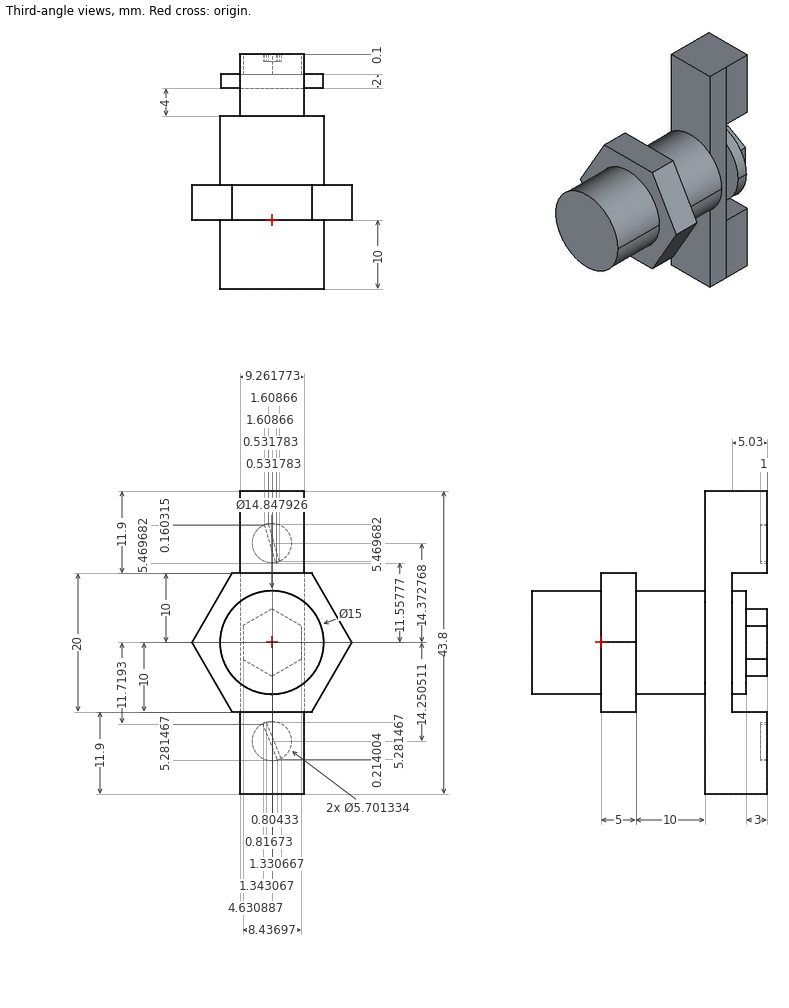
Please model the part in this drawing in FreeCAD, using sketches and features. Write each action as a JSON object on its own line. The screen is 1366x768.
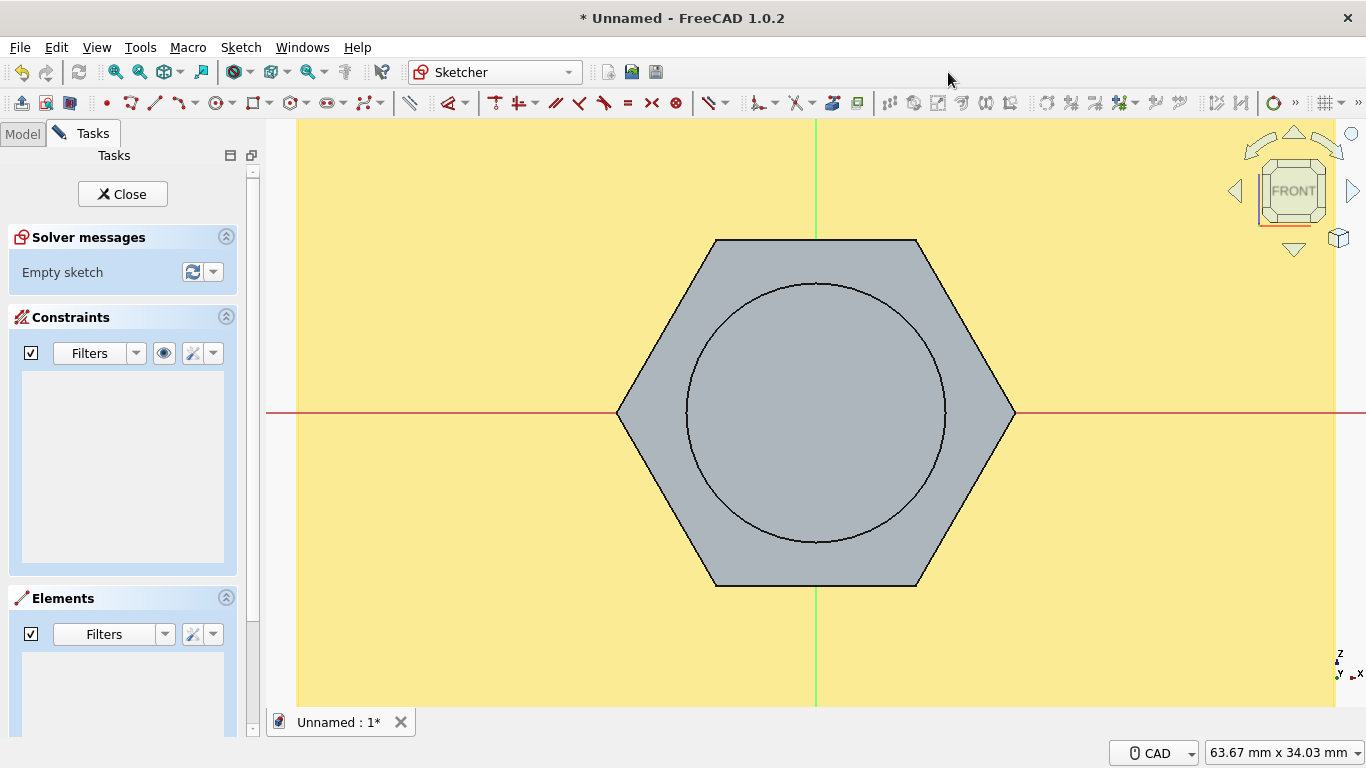
{"action": "left_click", "coordinate": [70, 104]}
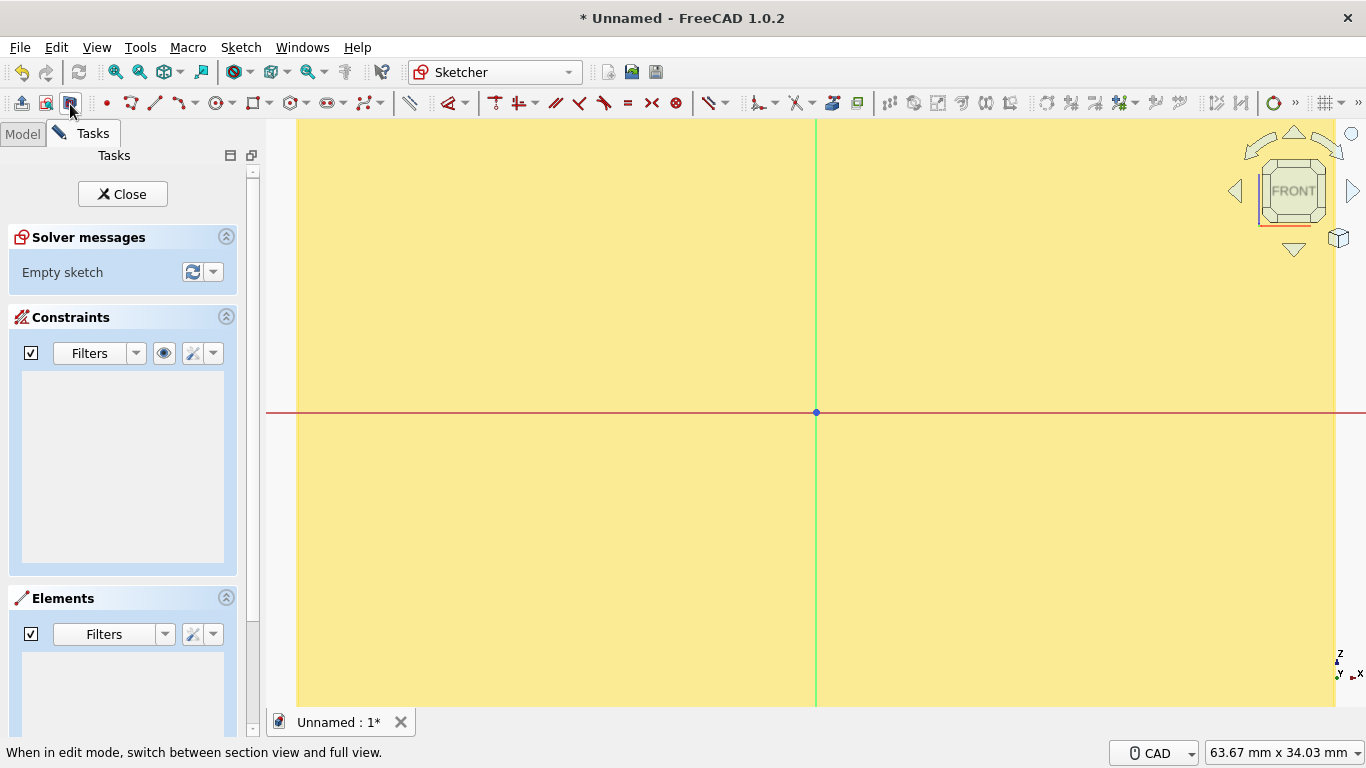
{"action": "scroll", "coordinate": [955, 413], "scroll_direction": "up", "scroll_amount": 2}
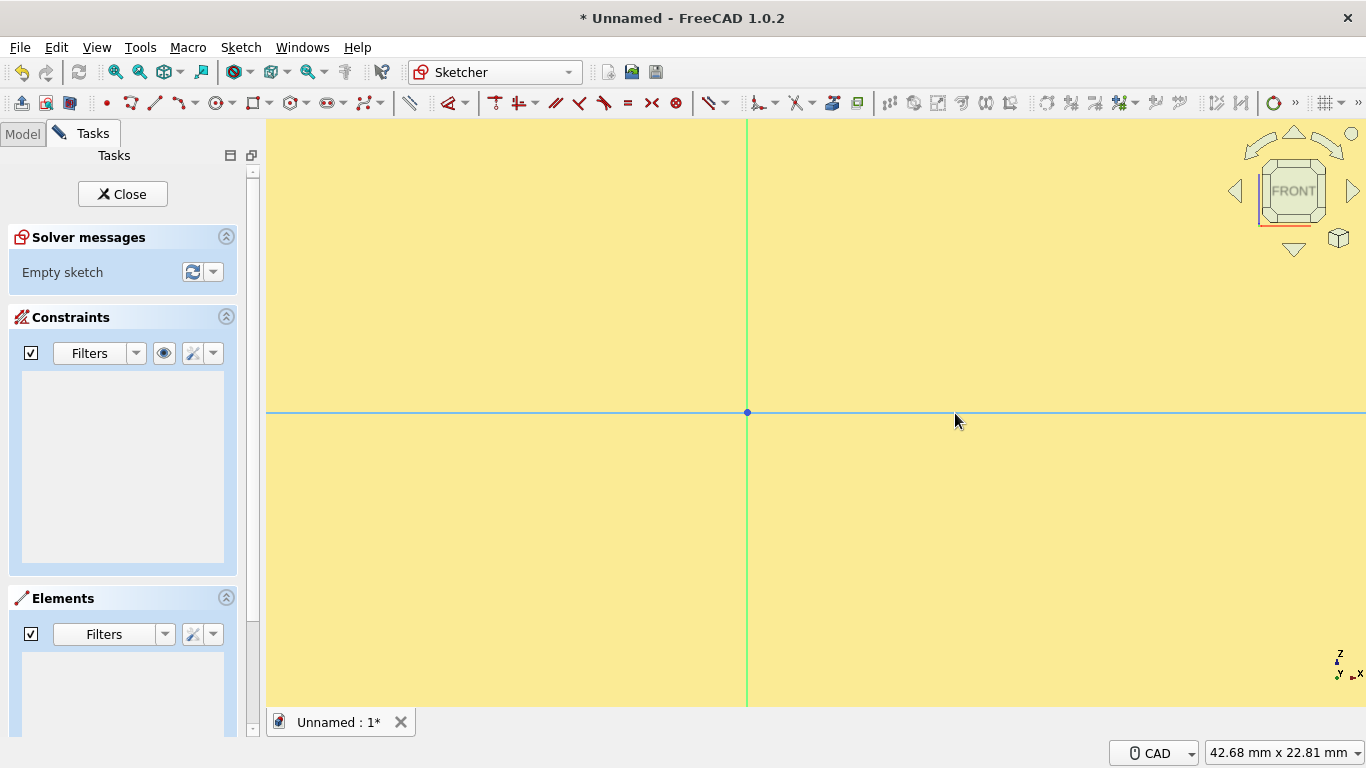
{"action": "left_click", "coordinate": [216, 104]}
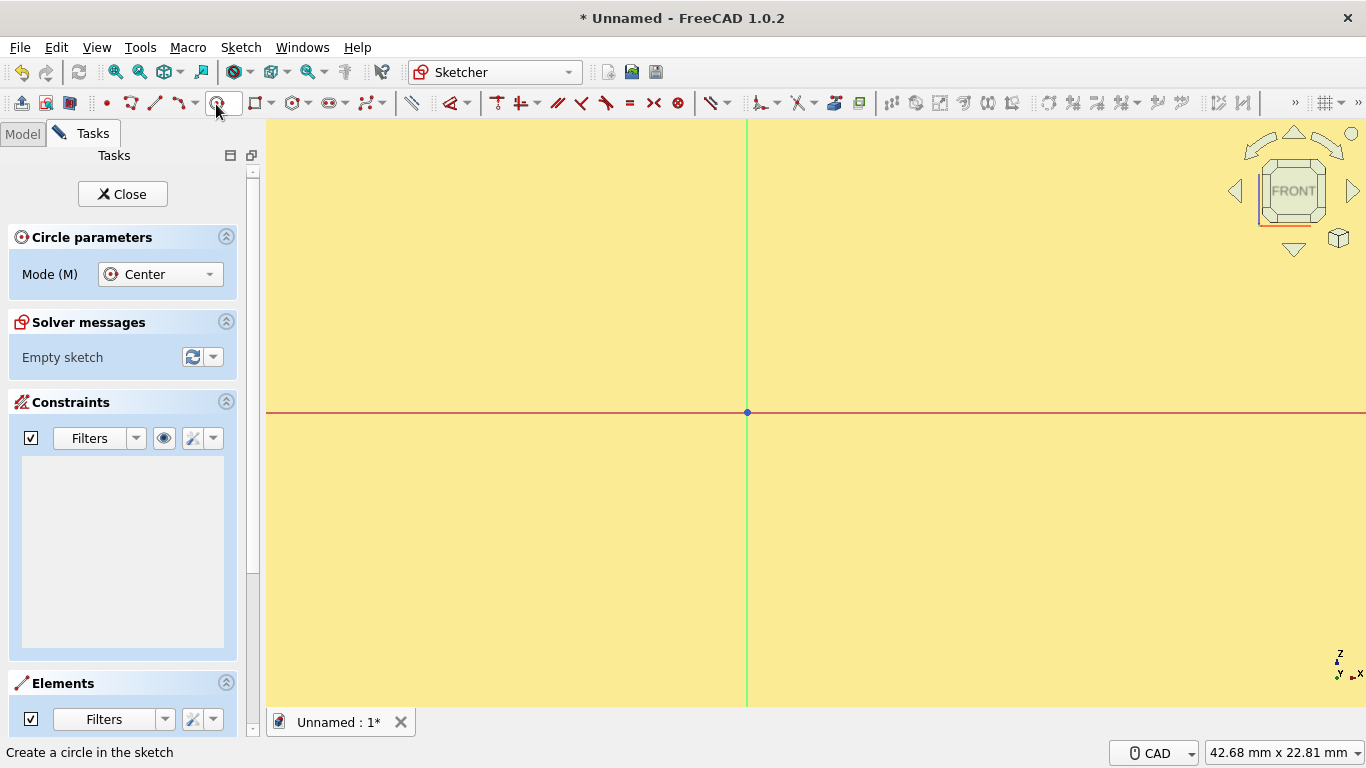
{"action": "left_click", "coordinate": [747, 413]}
{"action": "left_click", "coordinate": [884, 276]}
{"action": "key", "text": "Escape"}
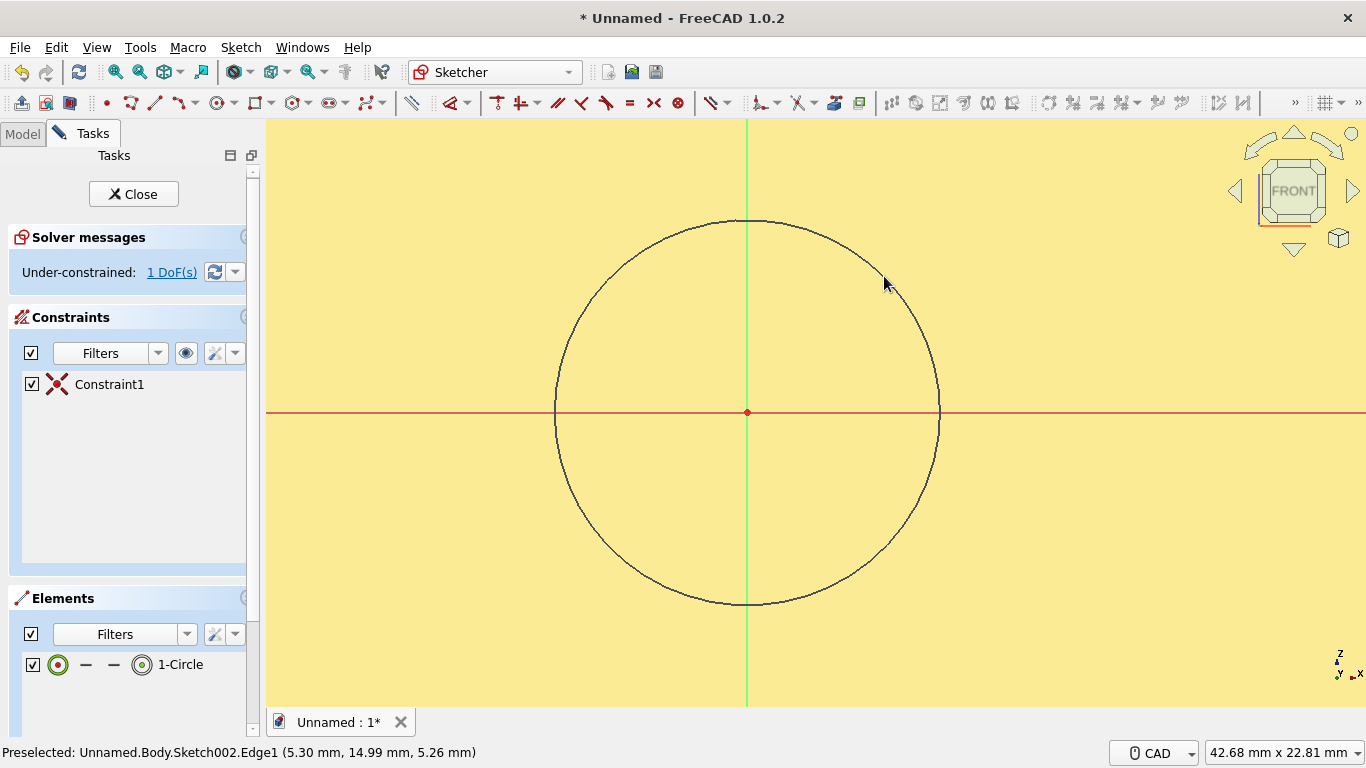
{"action": "left_click", "coordinate": [450, 104]}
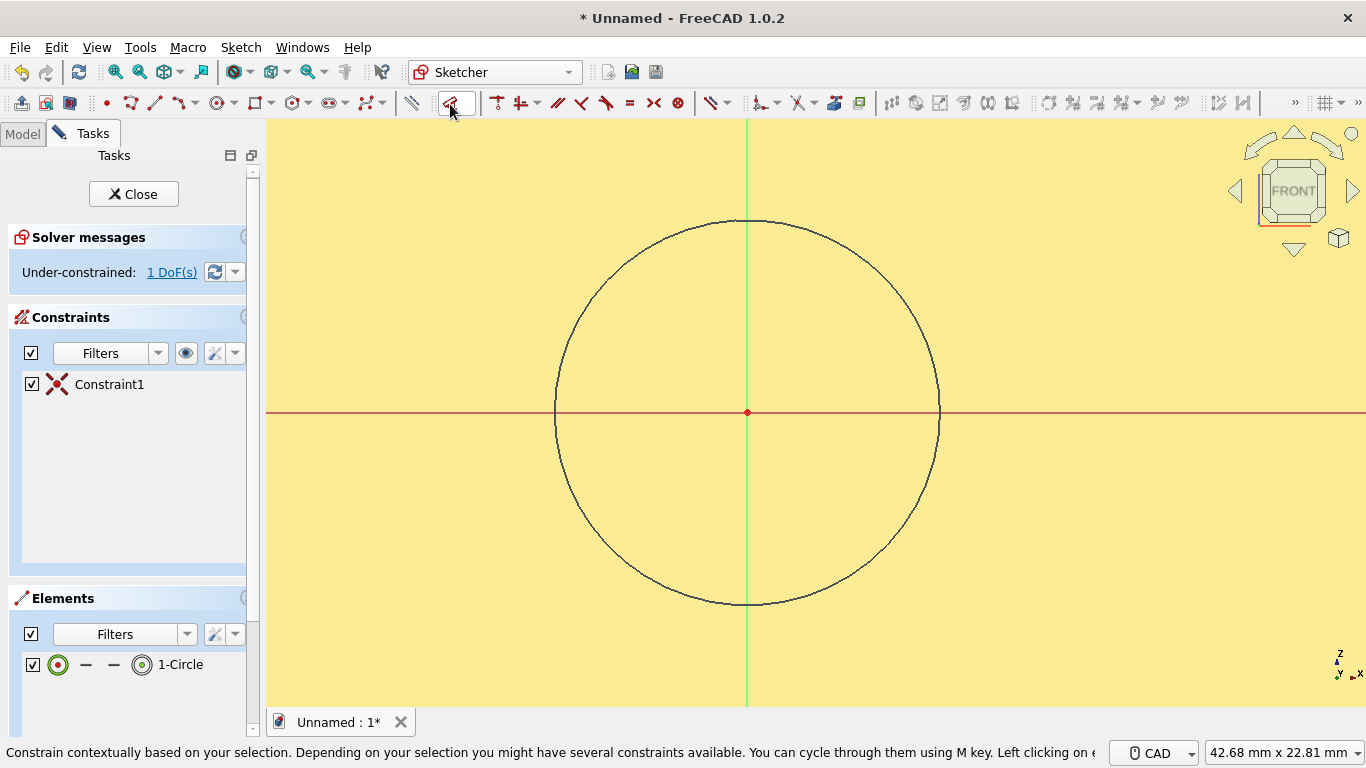
{"action": "left_click", "coordinate": [883, 276]}
{"action": "left_click", "coordinate": [906, 253]}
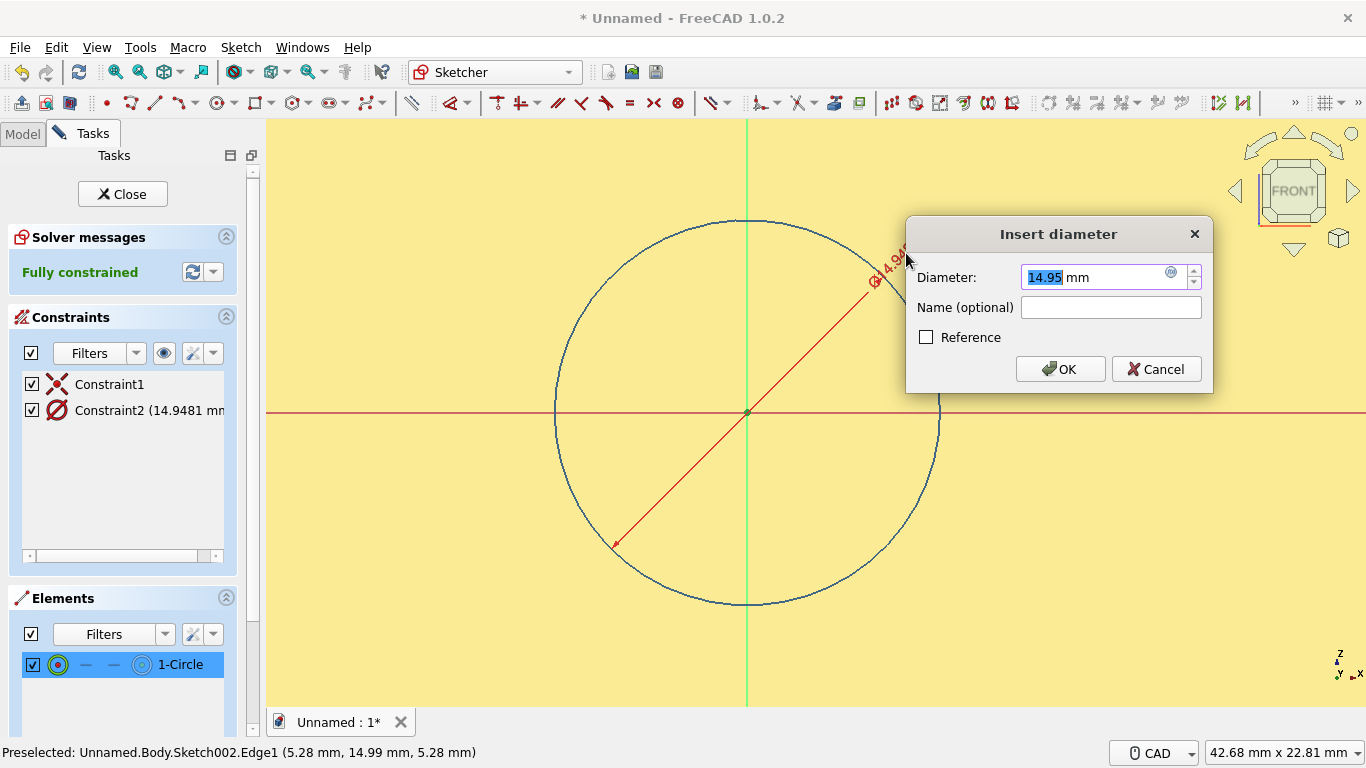
{"action": "type", "text": "15"}
{"action": "key", "text": "Return"}
{"action": "key", "text": "Escape"}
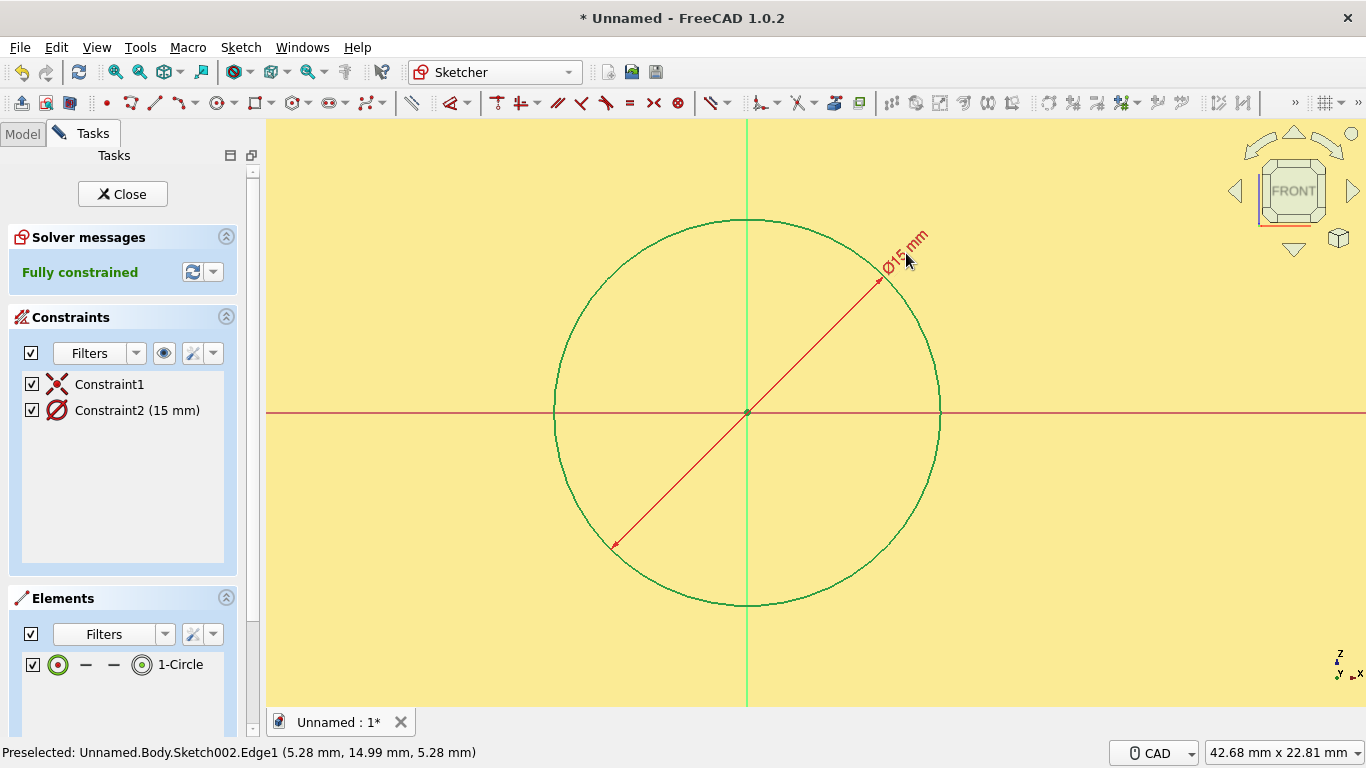
{"action": "left_click", "coordinate": [123, 194]}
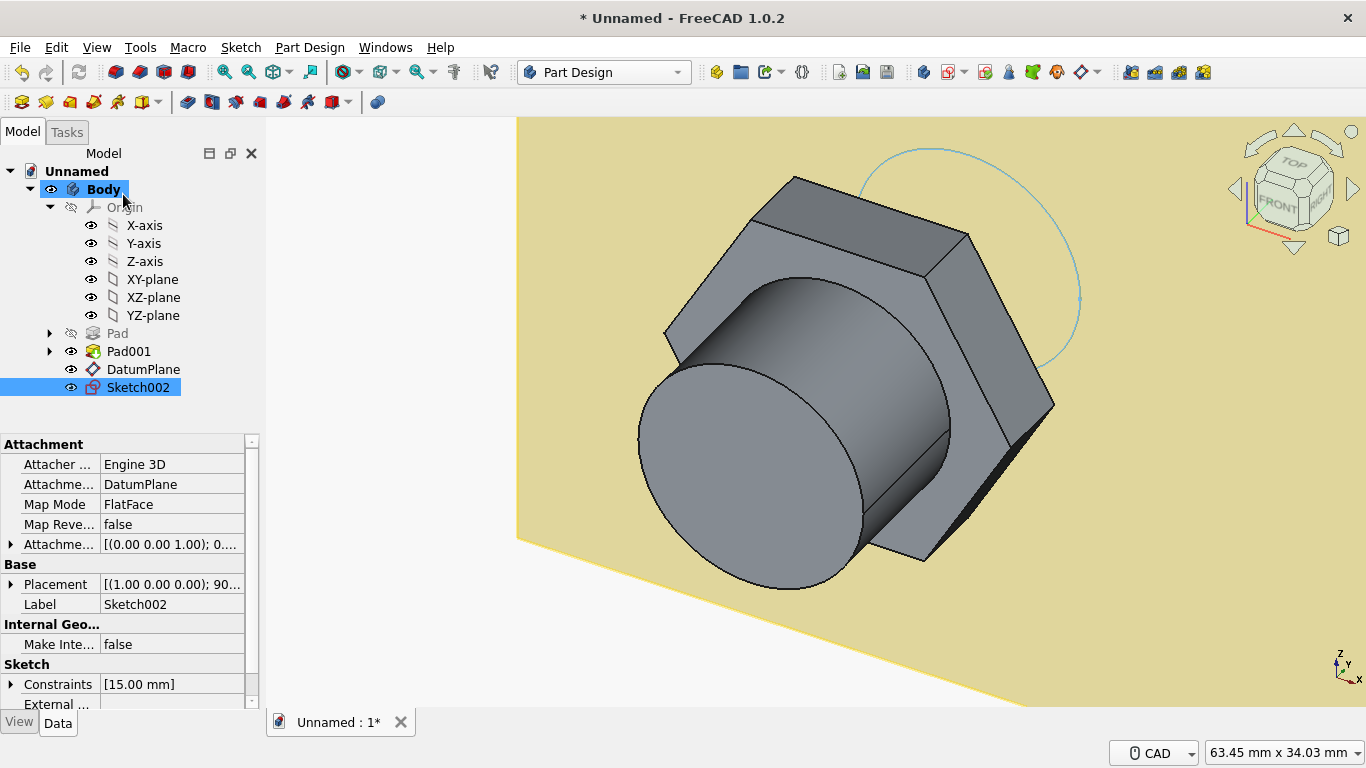
{"action": "left_click", "coordinate": [22, 102]}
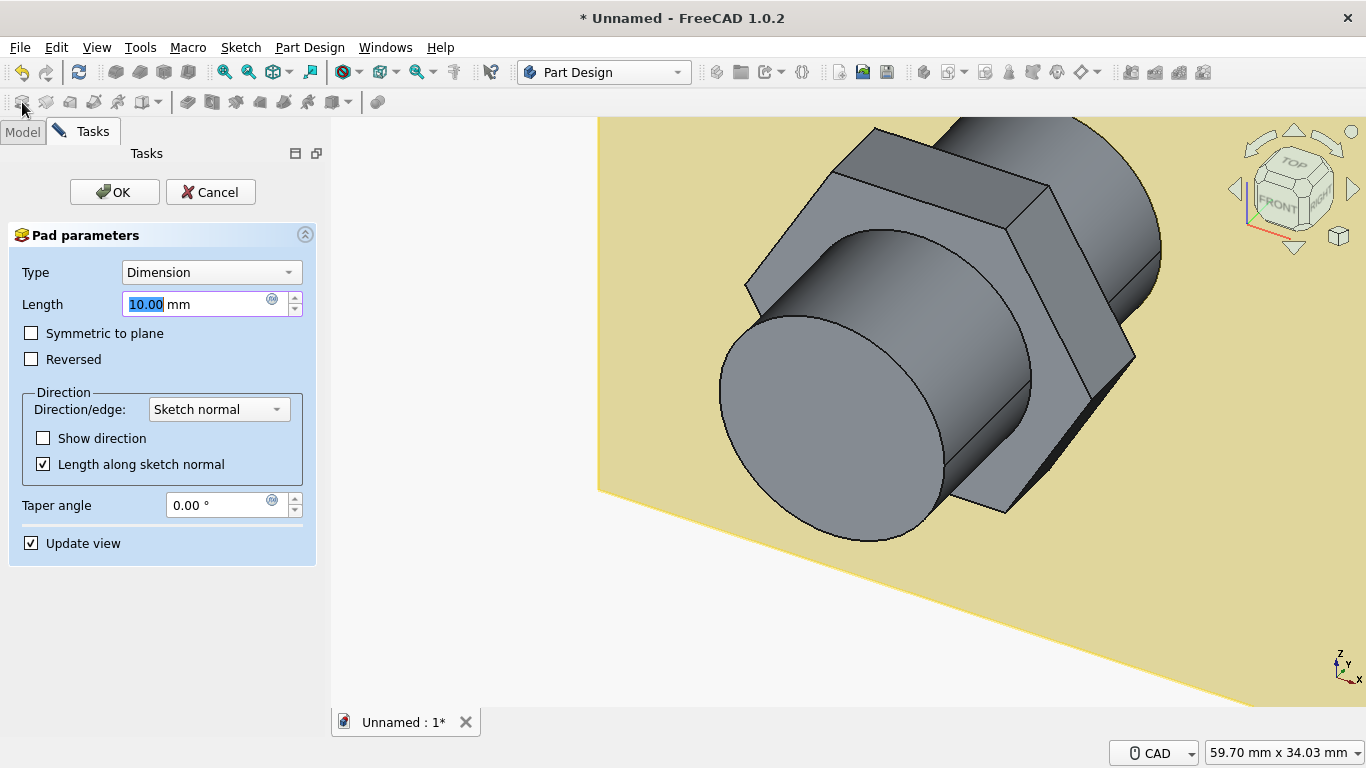
{"action": "type", "text": "10"}
{"action": "key", "text": "Tab"}